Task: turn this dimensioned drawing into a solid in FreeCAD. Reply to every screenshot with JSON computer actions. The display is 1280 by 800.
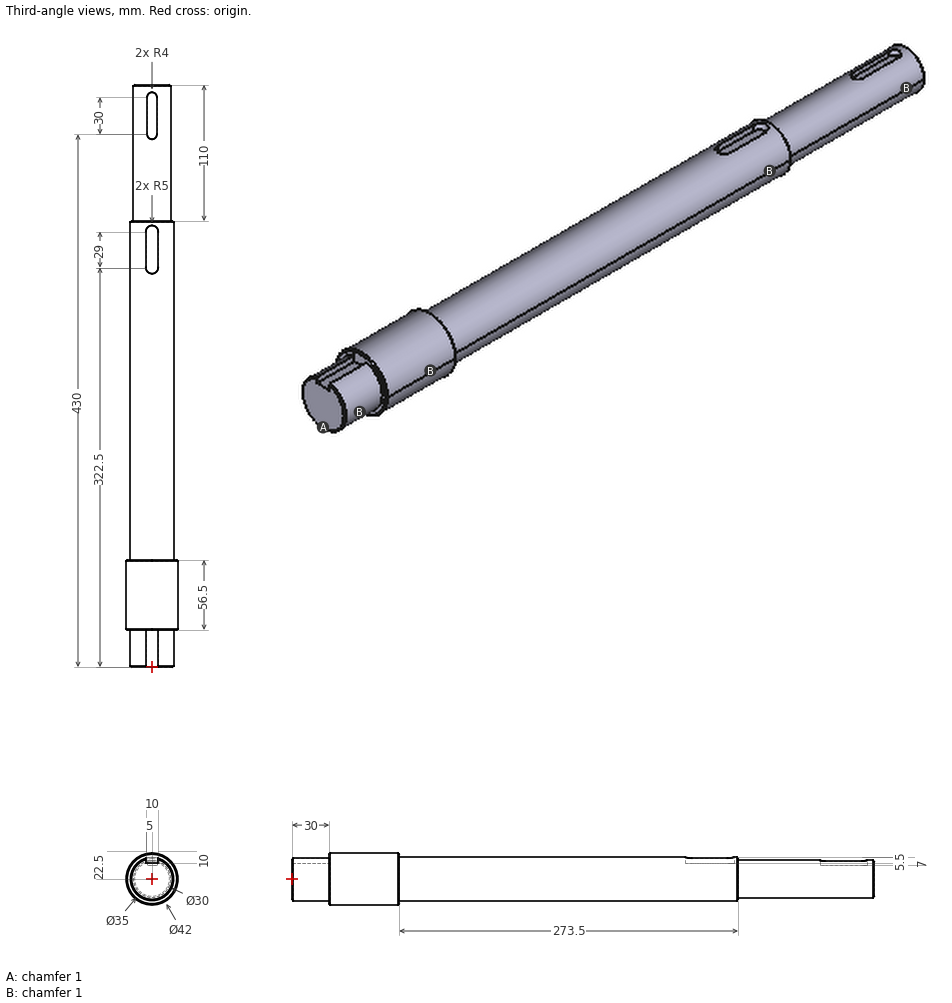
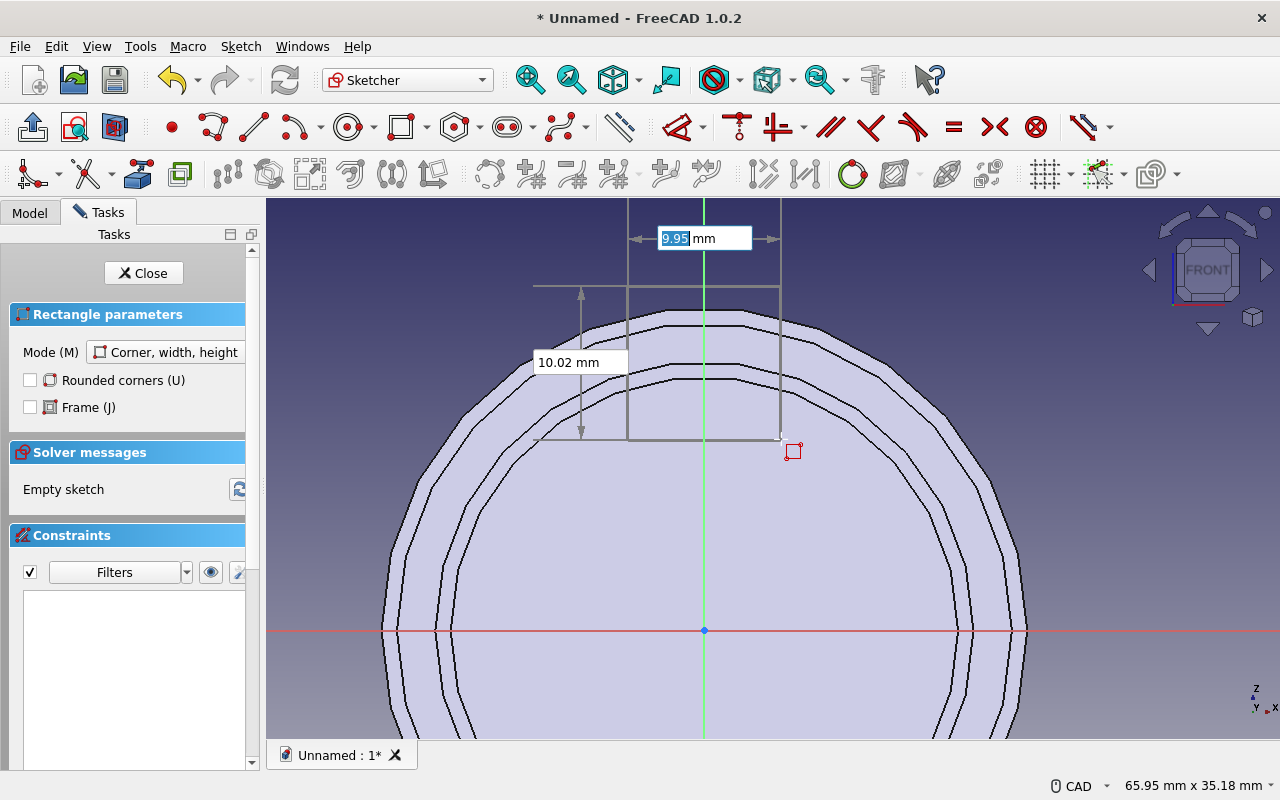
{"action": "type", "text": "10"}
{"action": "key", "text": "Tab"}
{"action": "type", "text": "10"}
{"action": "key", "text": "Return"}
{"action": "key", "text": "Escape"}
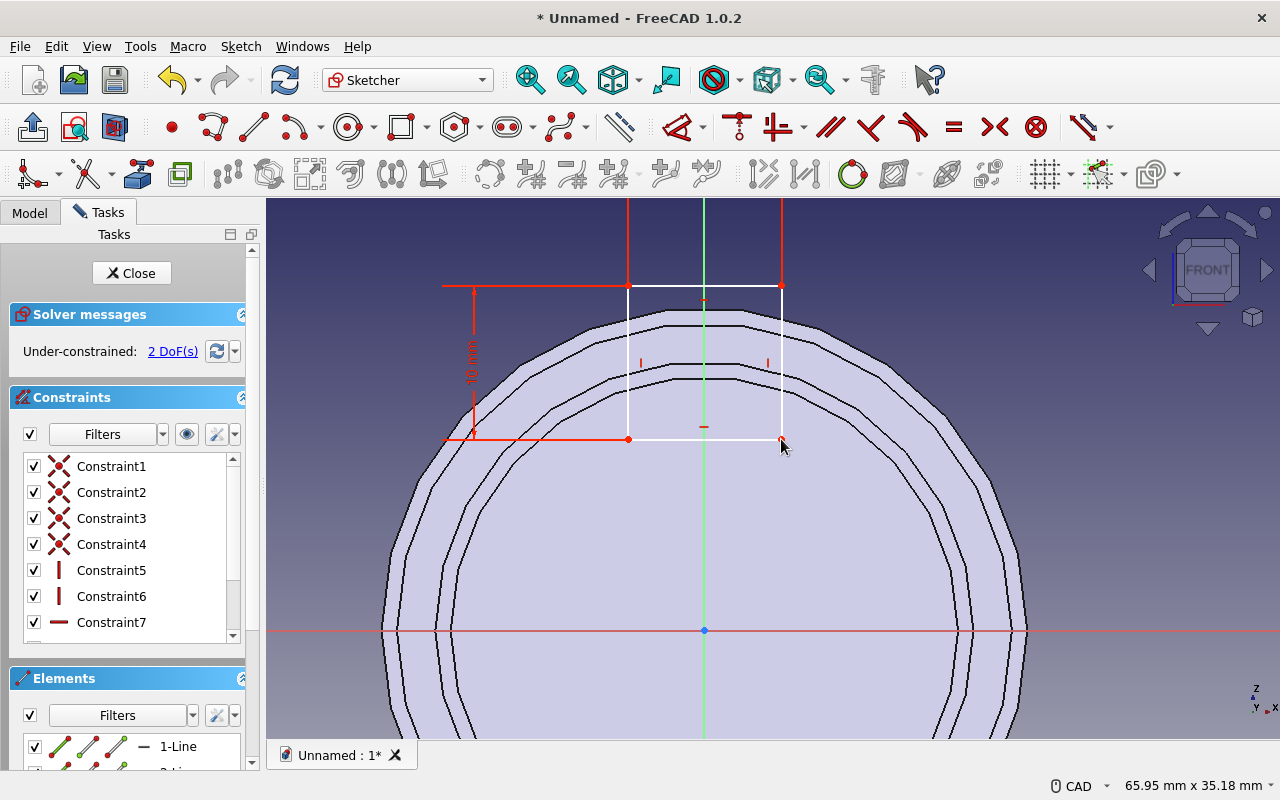
{"action": "left_click", "coordinate": [676, 128]}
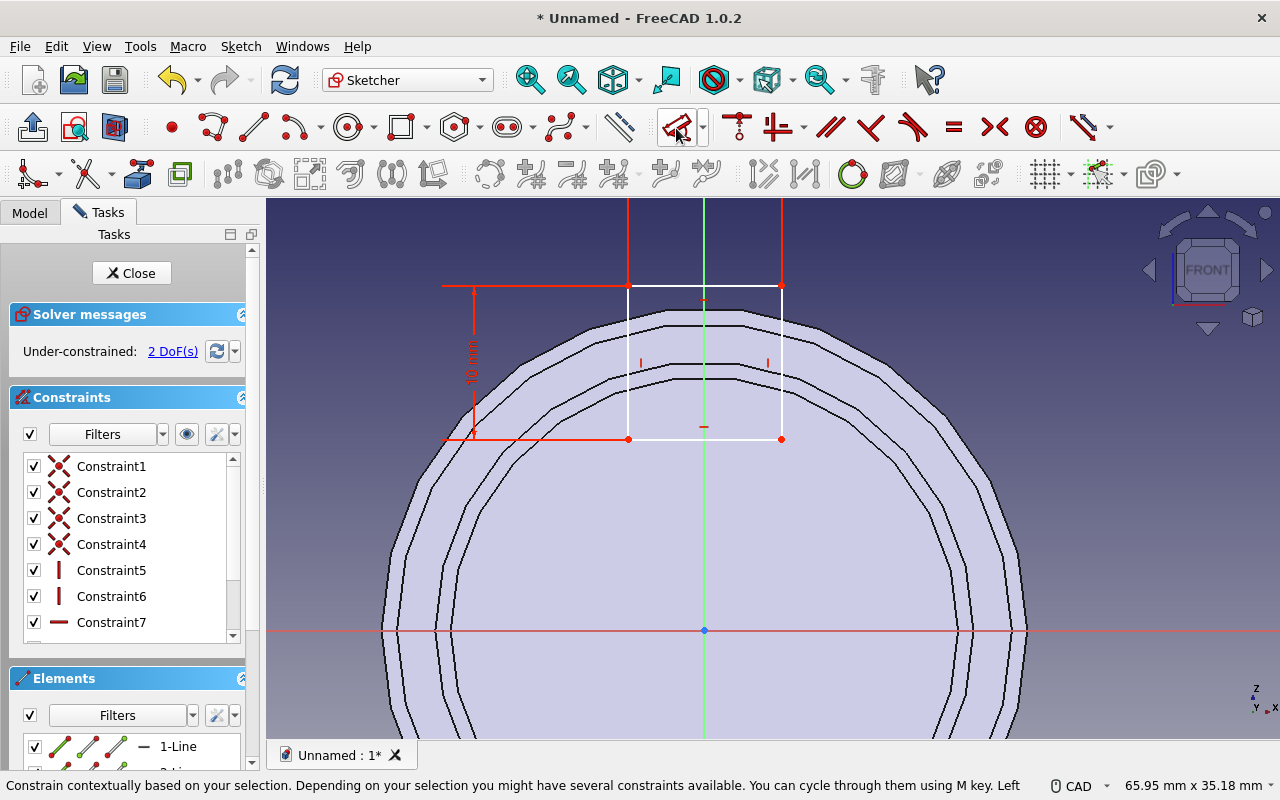
{"action": "left_click", "coordinate": [628, 286]}
{"action": "left_click", "coordinate": [666, 665]}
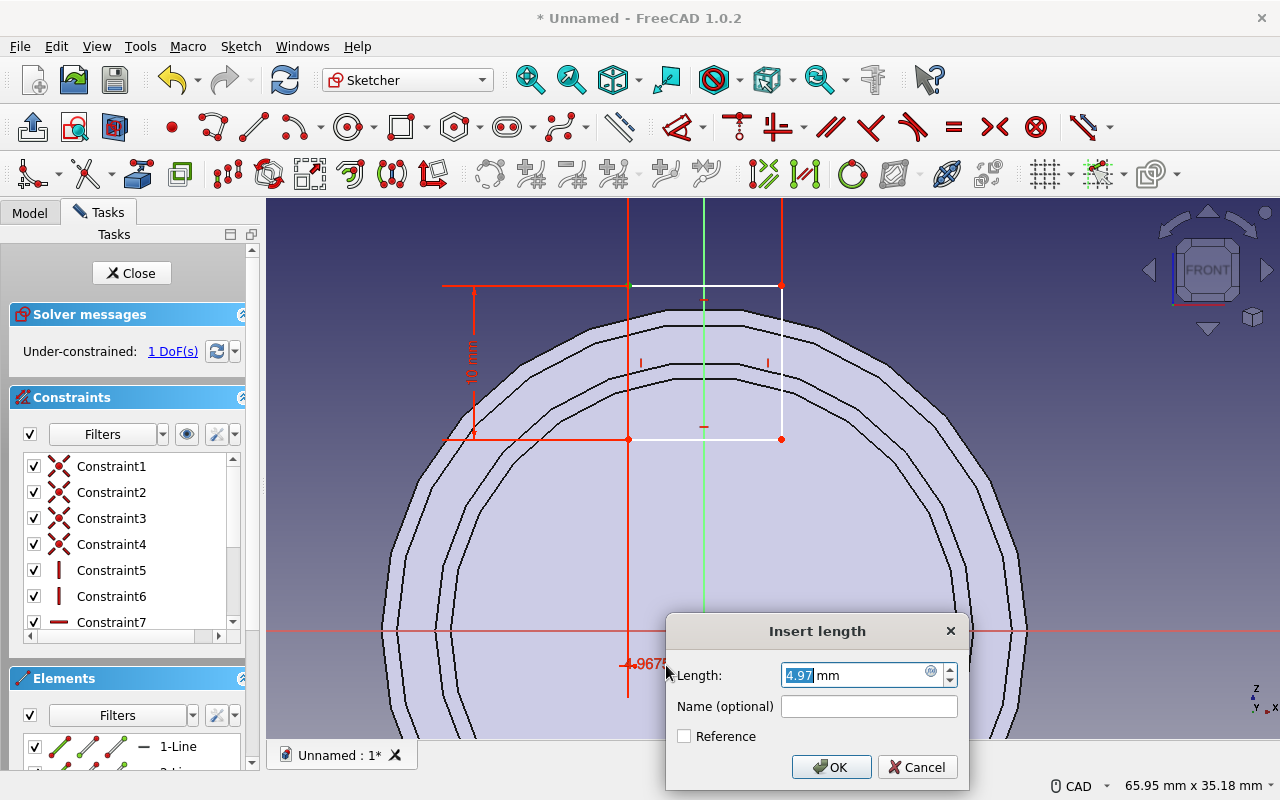
{"action": "type", "text": "5"}
{"action": "key", "text": "Return"}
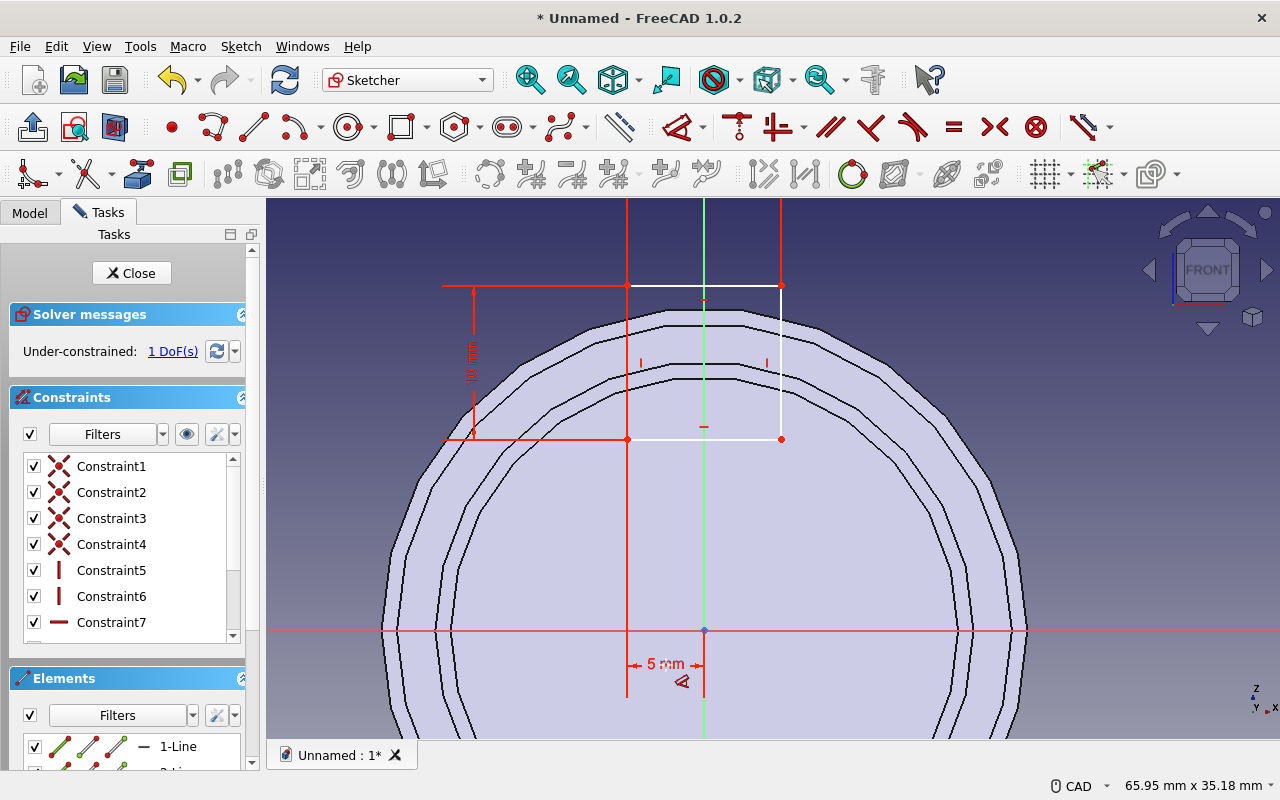
{"action": "left_click", "coordinate": [628, 286]}
{"action": "left_click", "coordinate": [594, 458]}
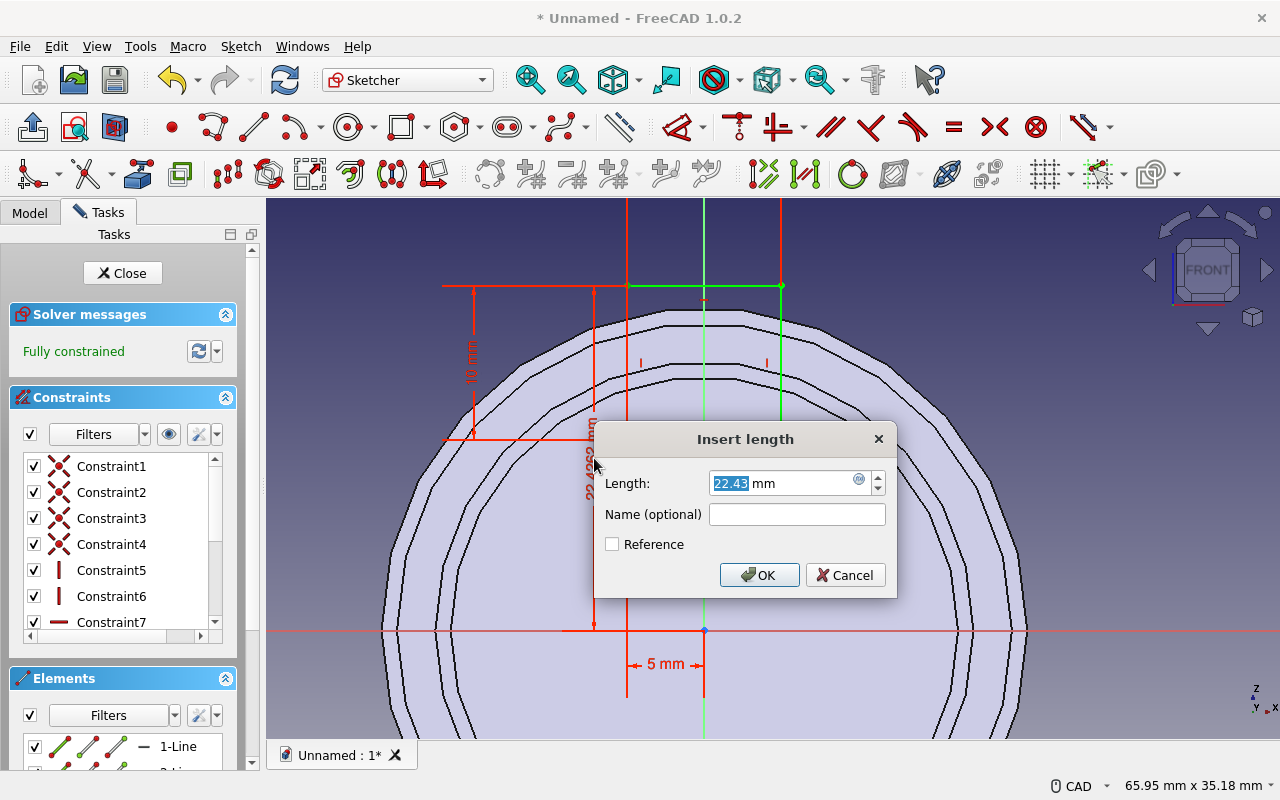
{"action": "type", "text": "22.5"}
{"action": "key", "text": "Return"}
{"action": "key", "text": "Escape"}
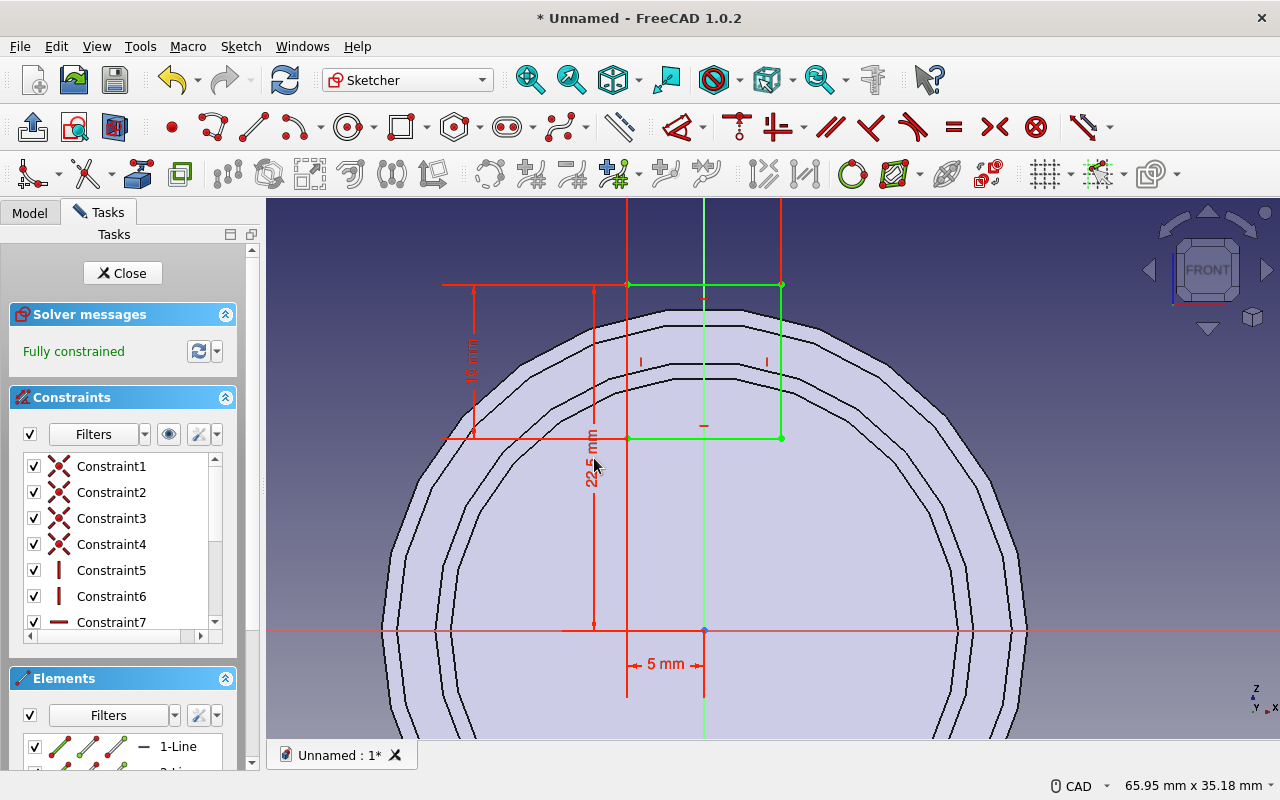
{"action": "left_click", "coordinate": [123, 273]}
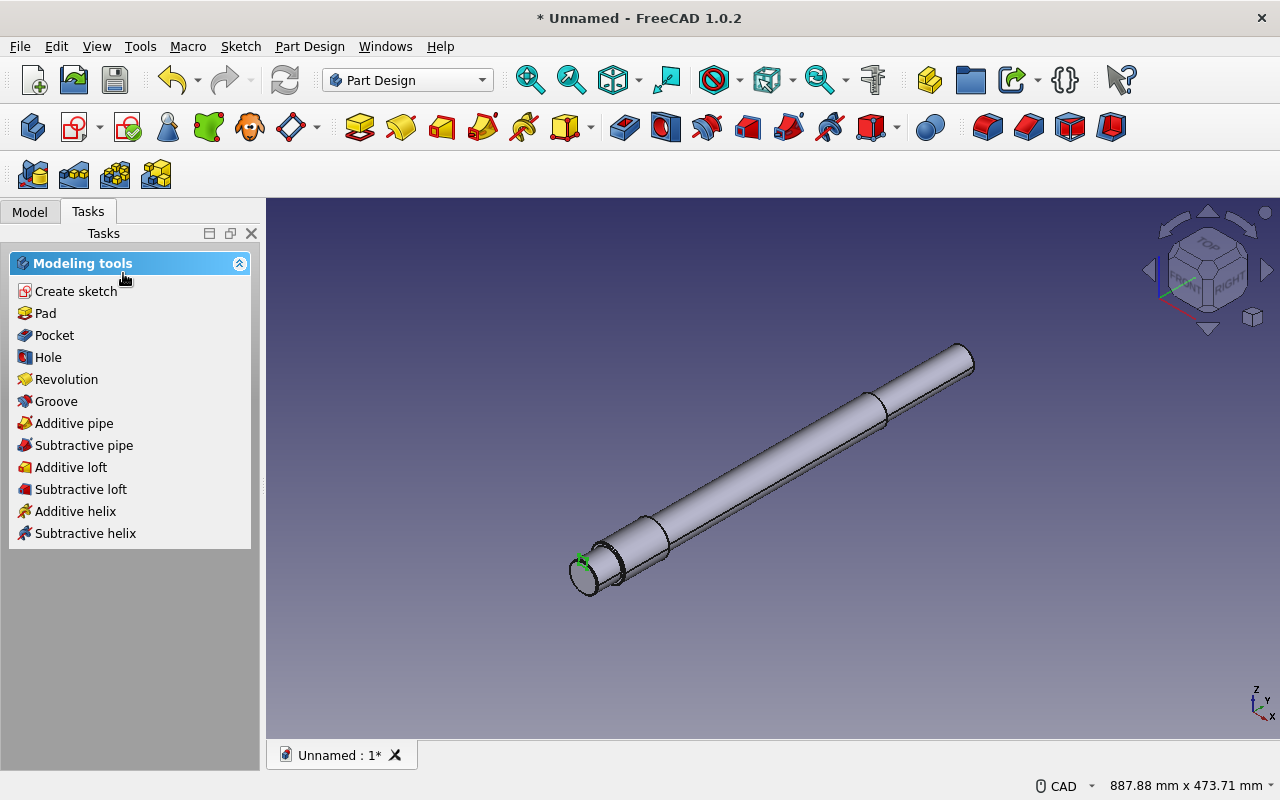
{"action": "left_click", "coordinate": [625, 128]}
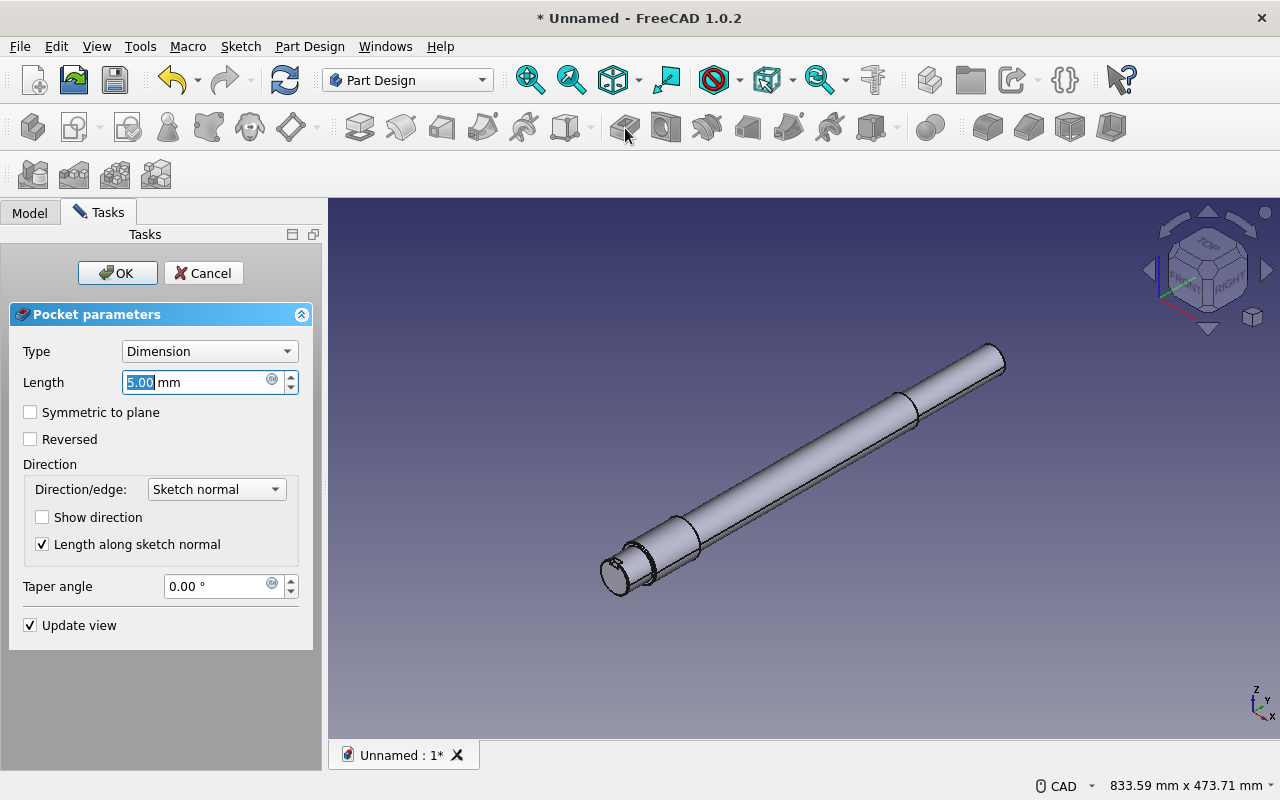
{"action": "type", "text": "30"}
{"action": "key", "text": "Tab"}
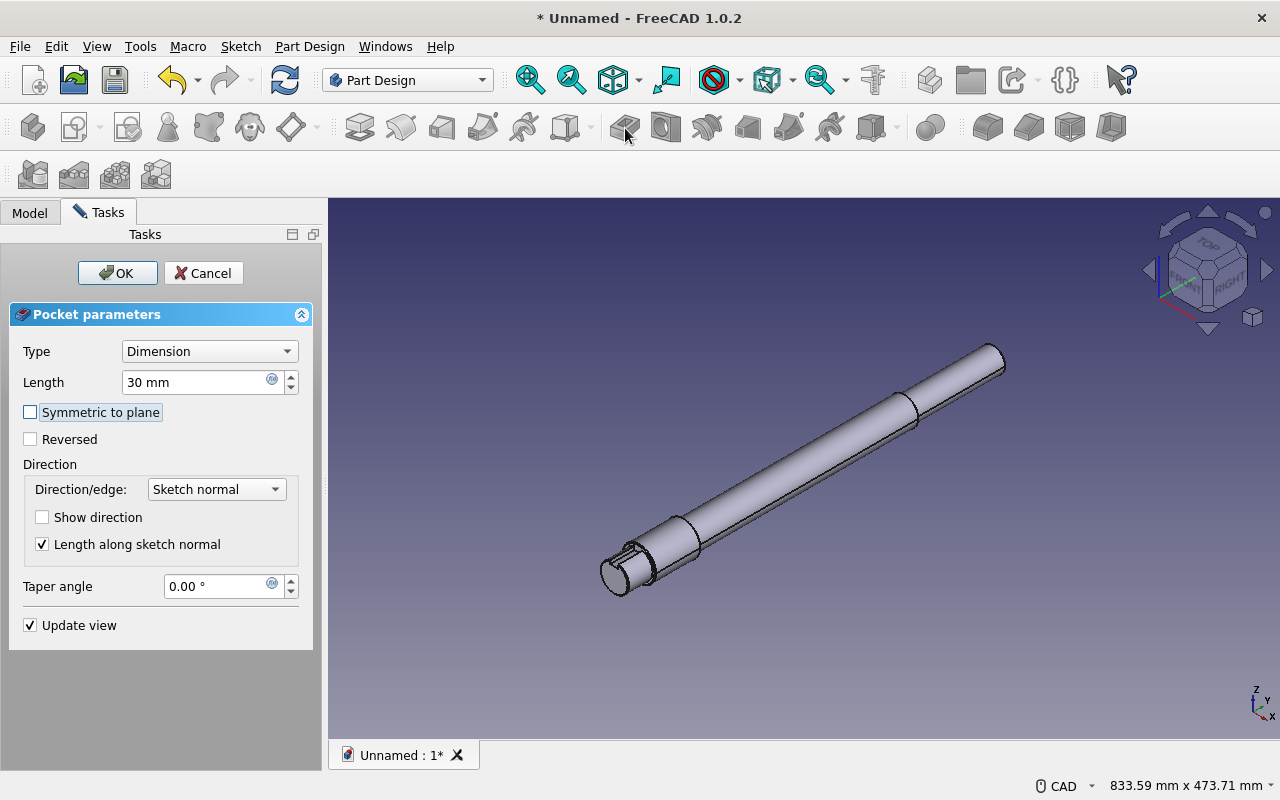
{"action": "left_click", "coordinate": [118, 273]}